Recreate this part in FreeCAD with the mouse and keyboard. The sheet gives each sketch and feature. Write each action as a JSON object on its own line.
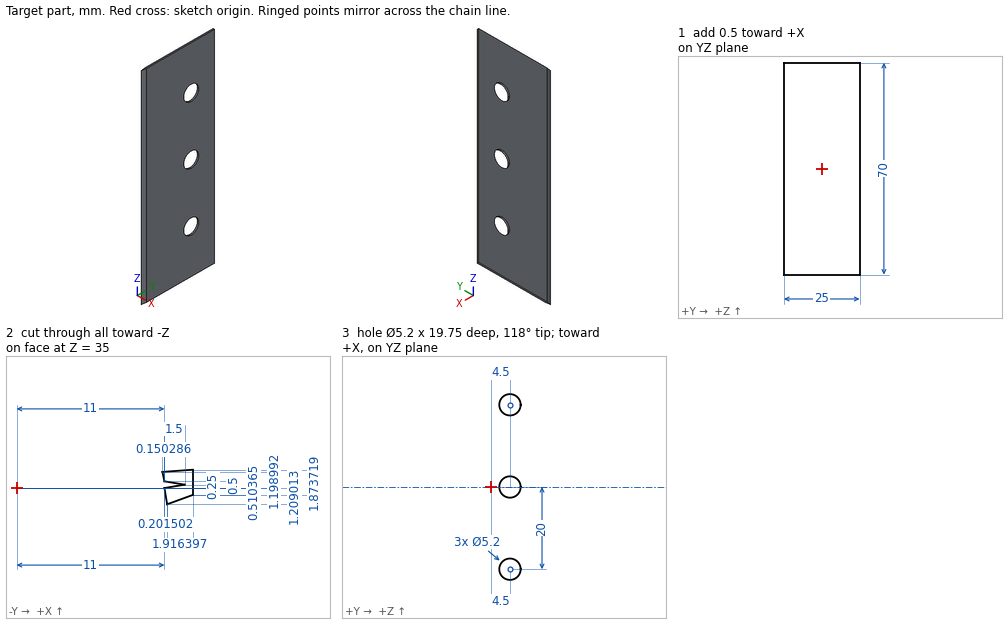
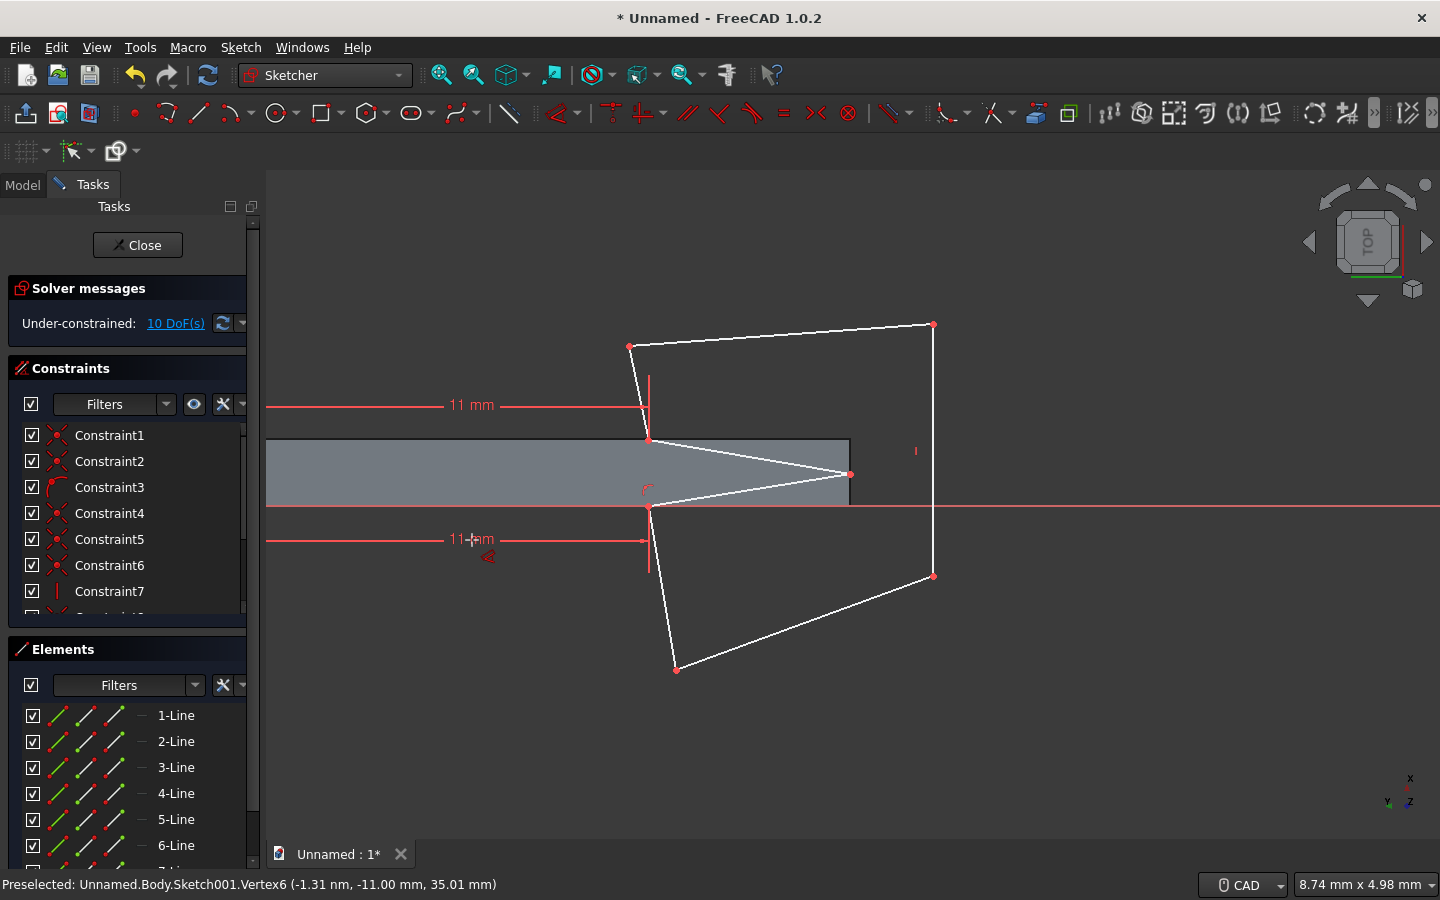
{"action": "left_click", "coordinate": [649, 440]}
{"action": "left_click", "coordinate": [683, 473]}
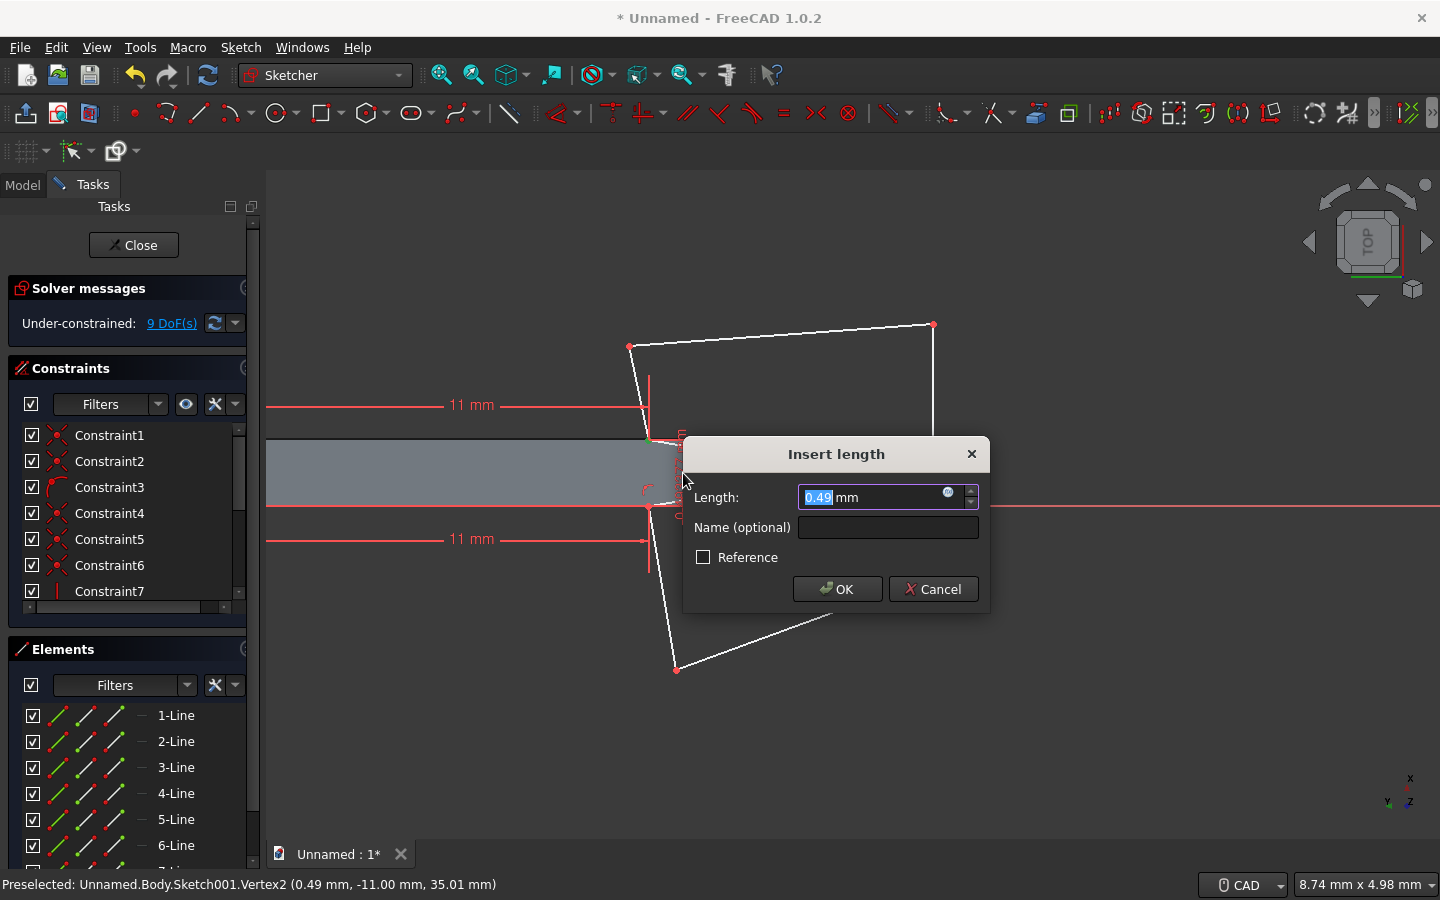
{"action": "type", "text": "0.5"}
{"action": "key", "text": "Return"}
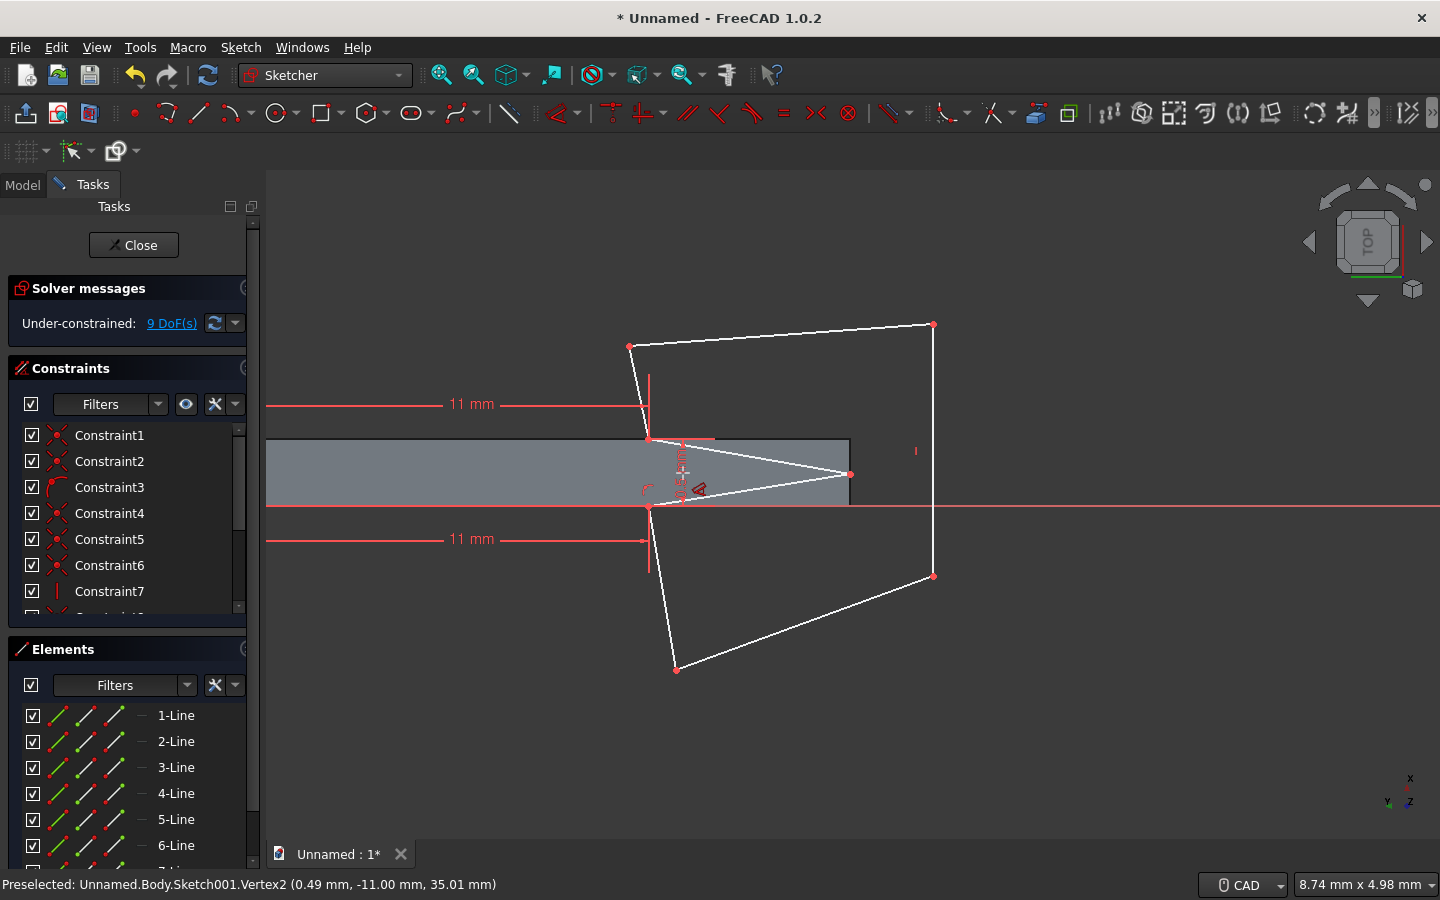
{"action": "left_click", "coordinate": [709, 450]}
{"action": "left_click", "coordinate": [749, 405]}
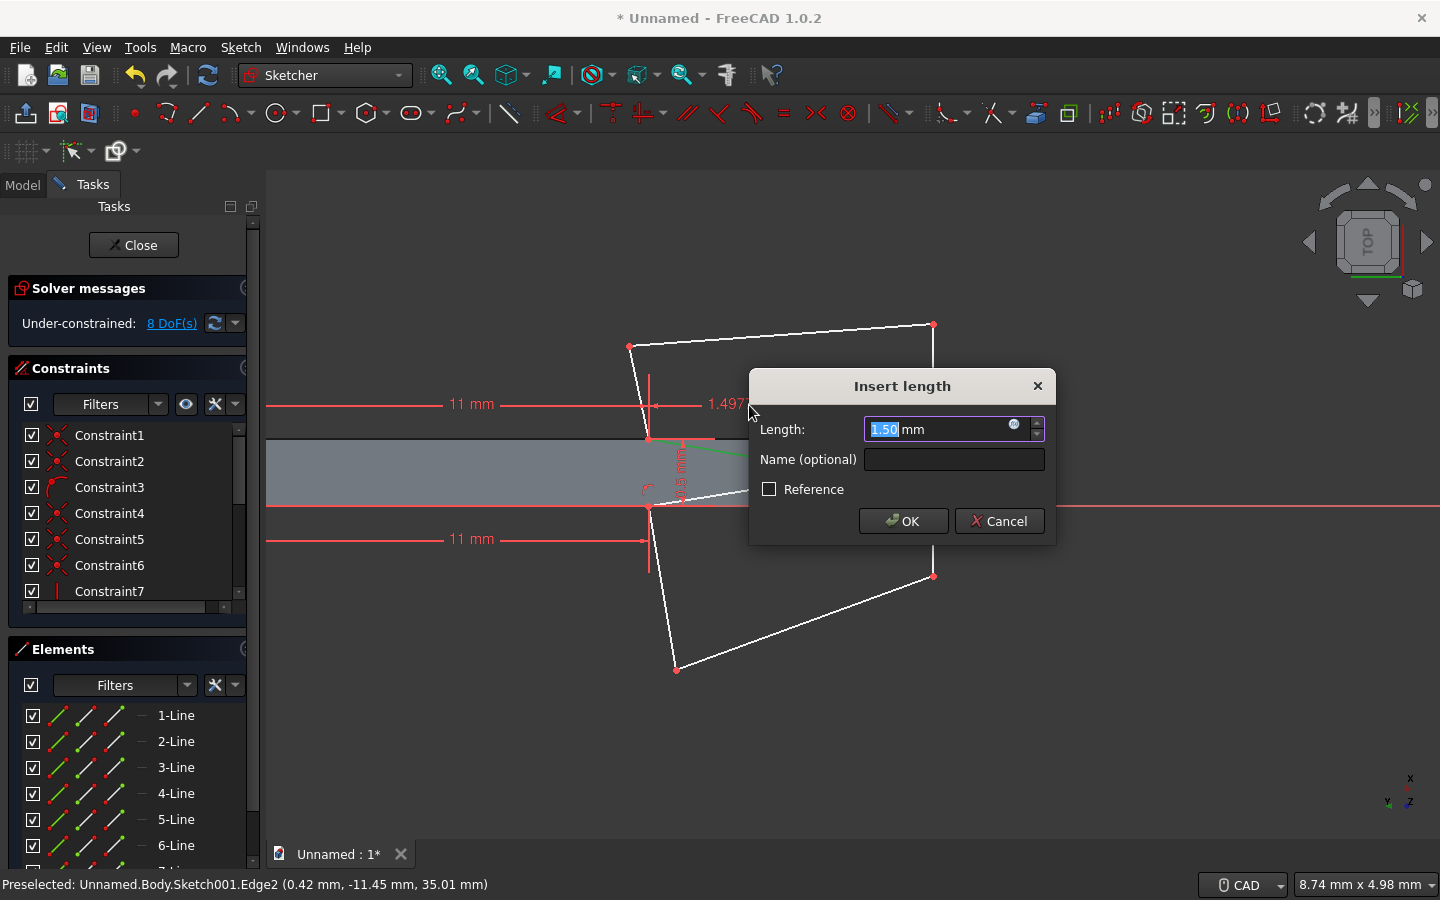
{"action": "type", "text": "1.5"}
{"action": "key", "text": "Return"}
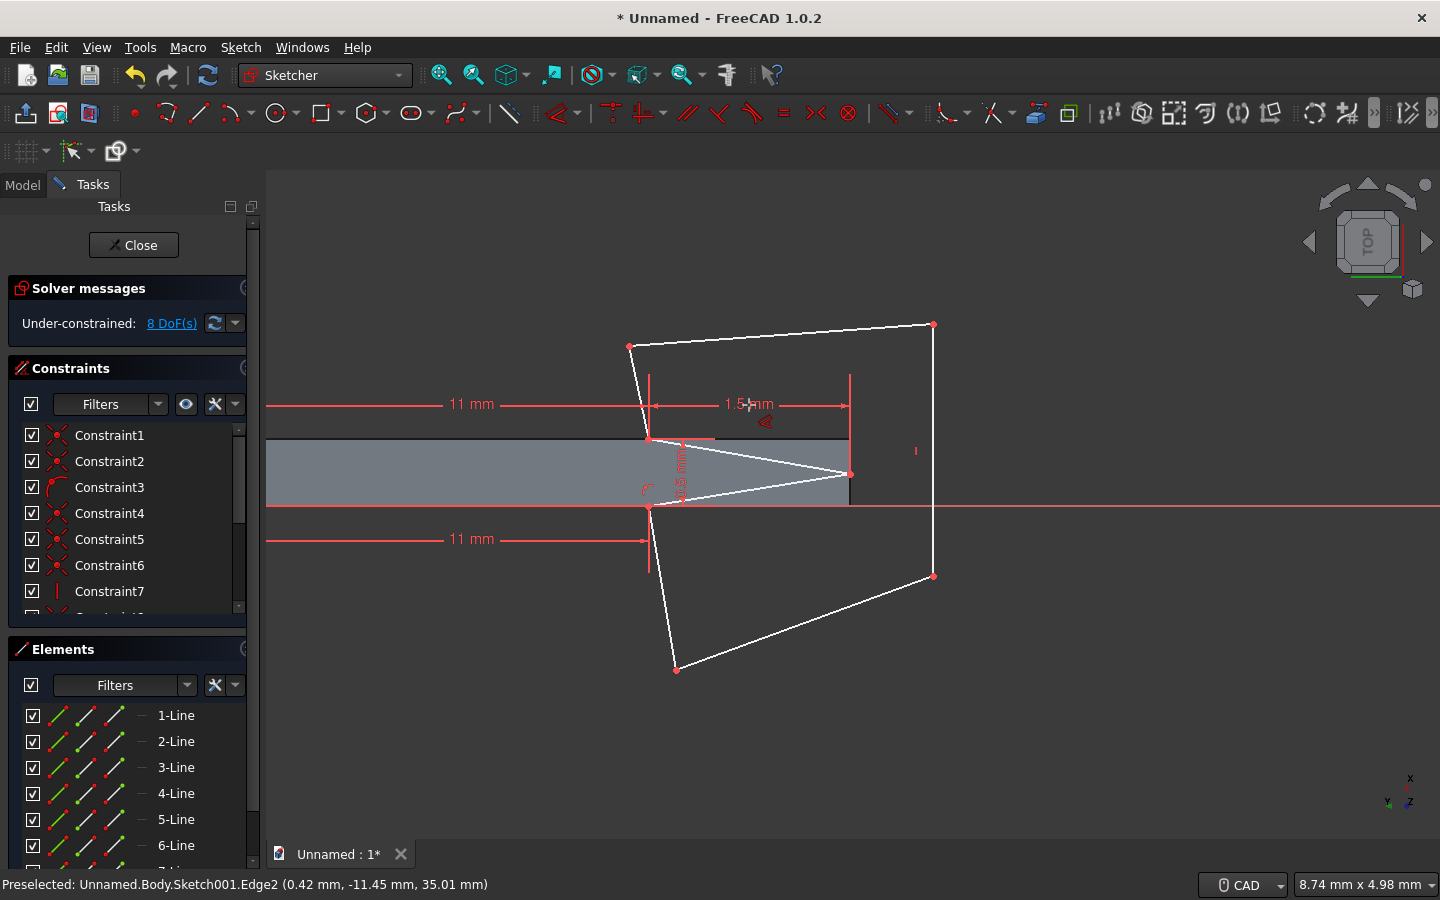
{"action": "left_click", "coordinate": [850, 474]}
{"action": "left_click", "coordinate": [884, 490]}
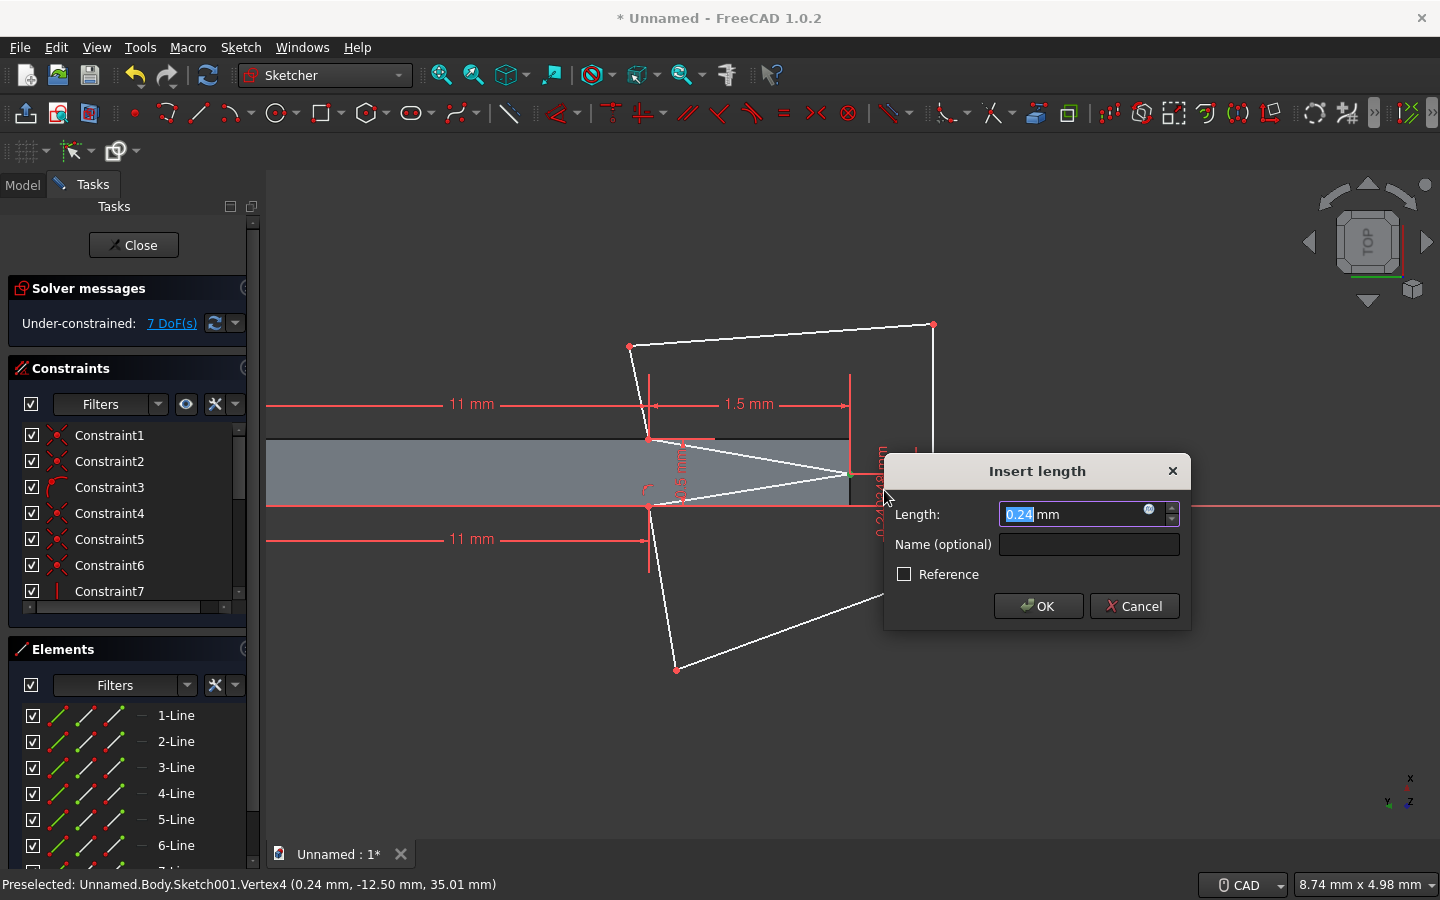
{"action": "type", "text": "0.25"}
{"action": "key", "text": "Return"}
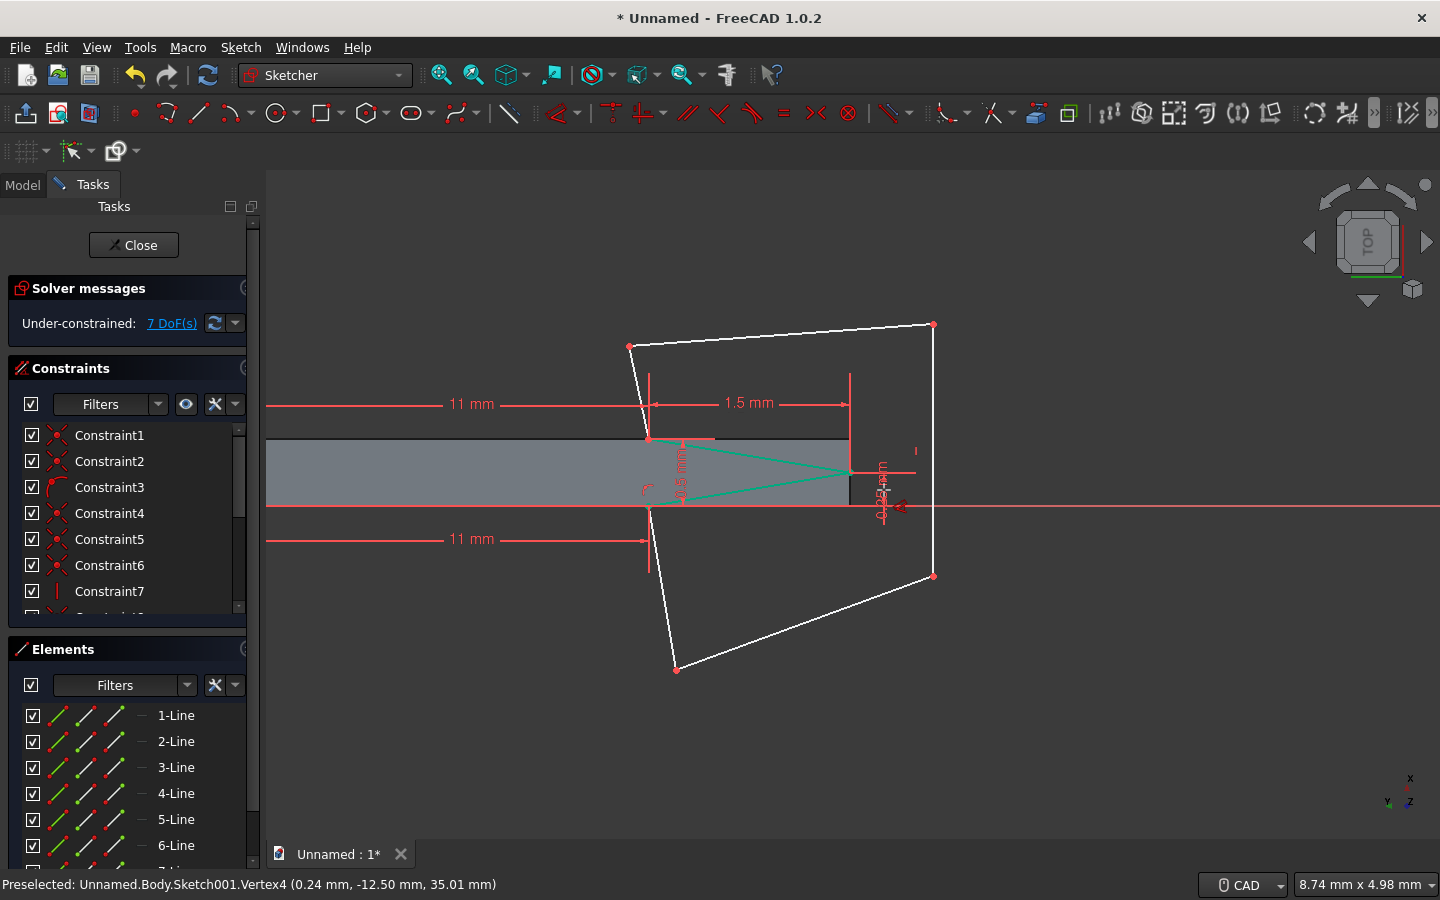
{"action": "left_click", "coordinate": [933, 400]}
{"action": "left_click", "coordinate": [967, 450]}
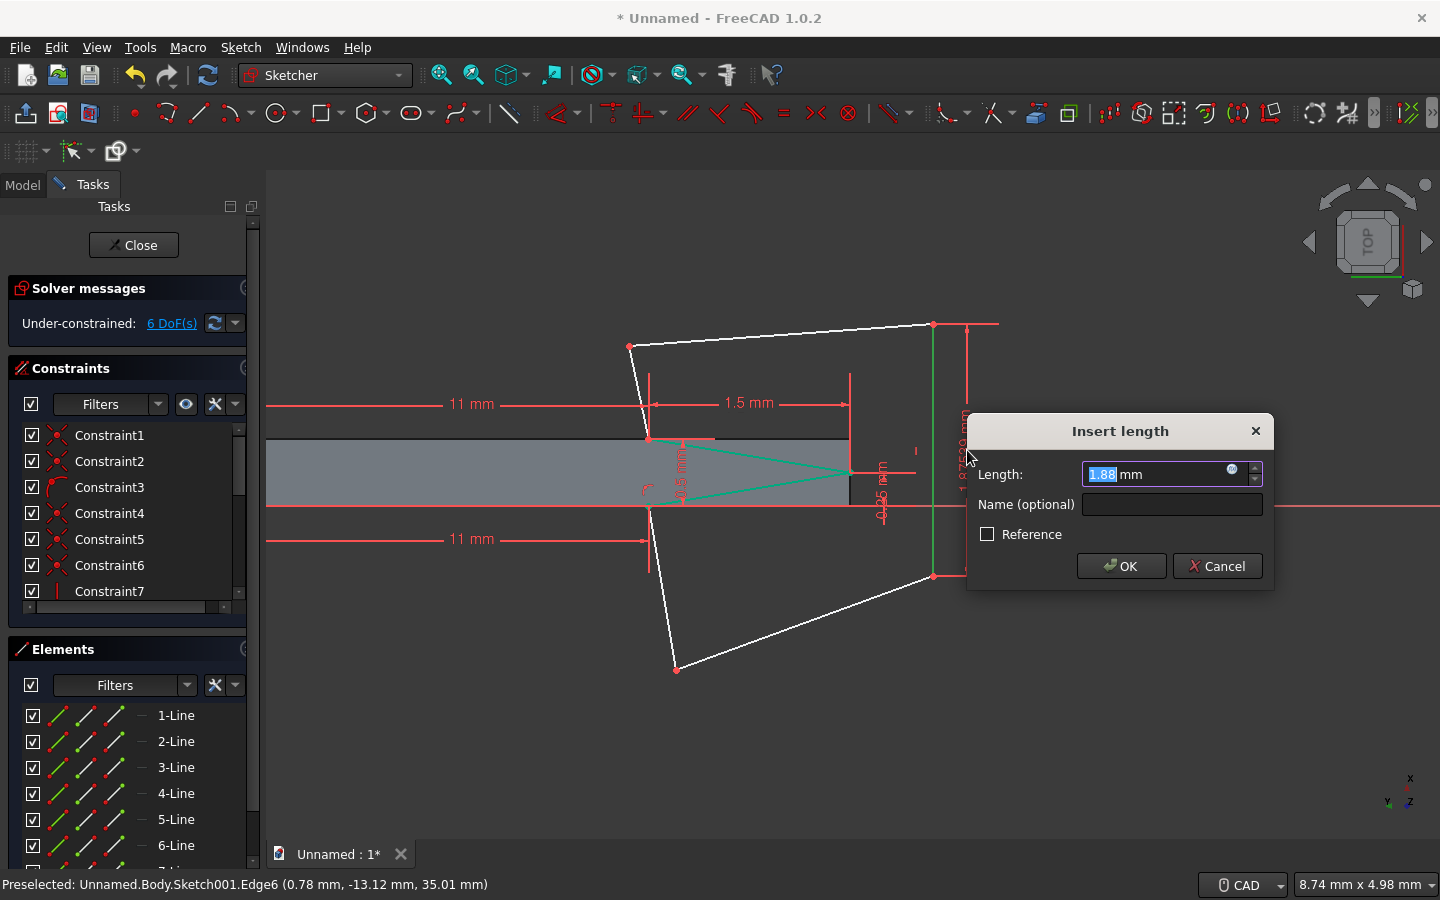
{"action": "type", "text": "1.873719"}
{"action": "key", "text": "Return"}